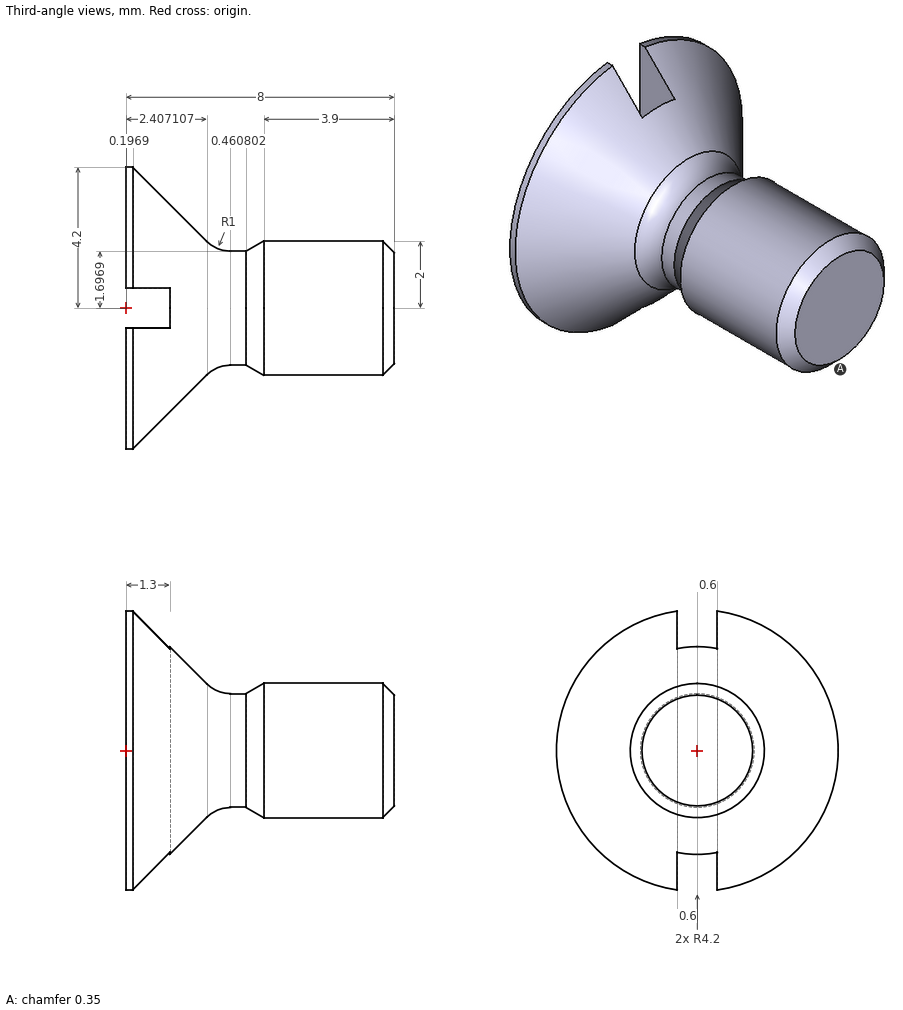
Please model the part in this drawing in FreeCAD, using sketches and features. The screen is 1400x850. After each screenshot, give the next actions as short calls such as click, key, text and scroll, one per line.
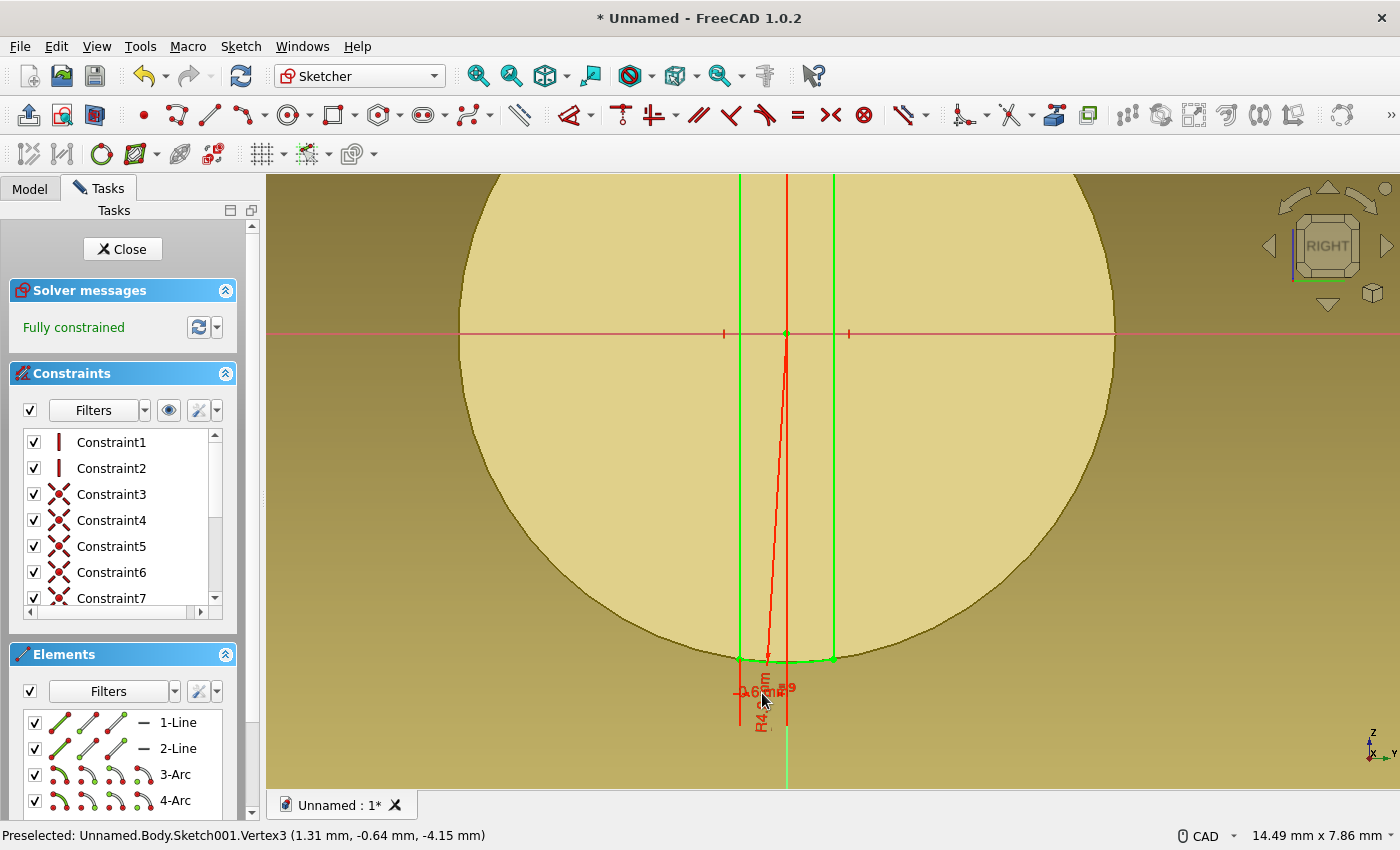
click(123, 249)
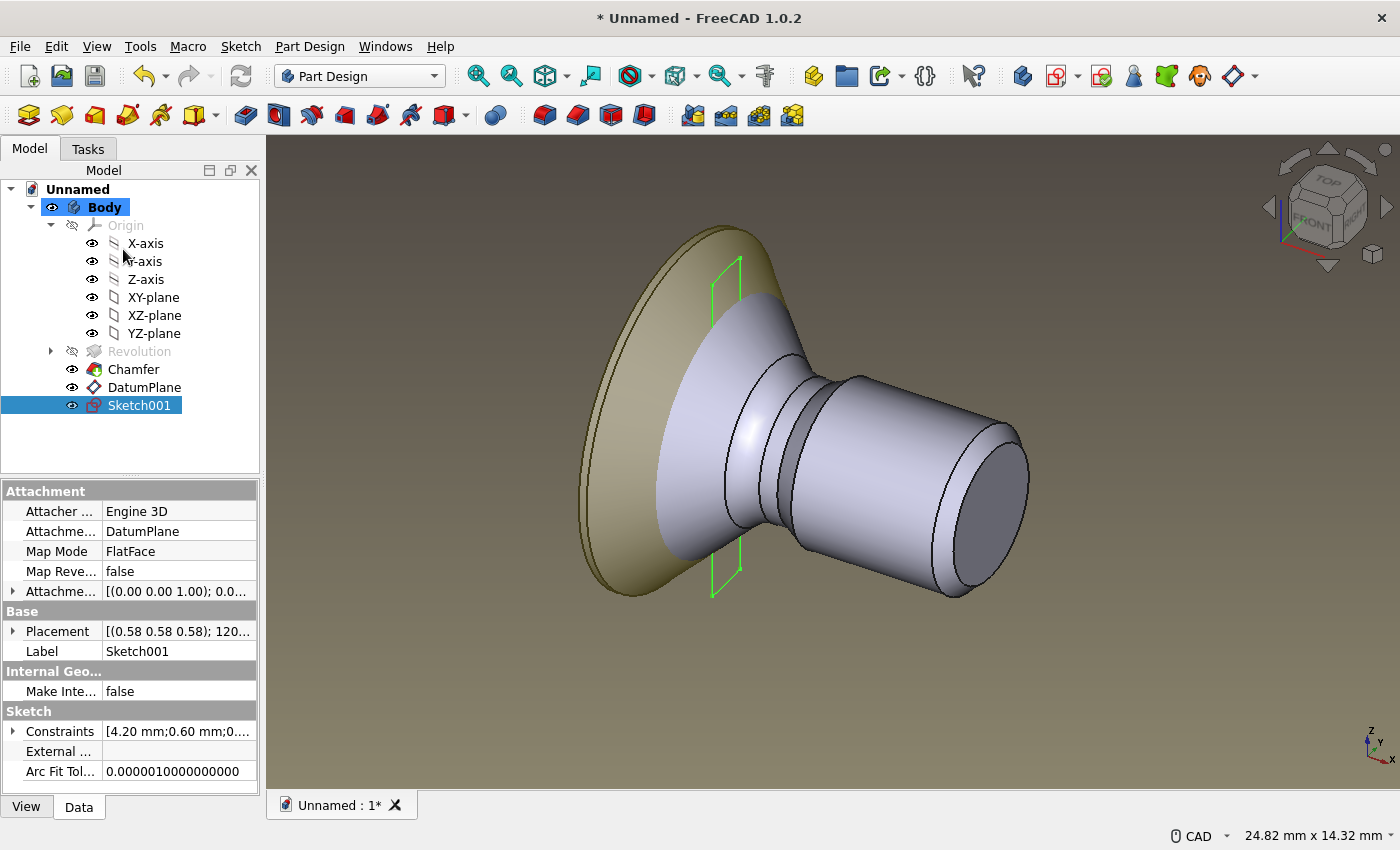
click(246, 116)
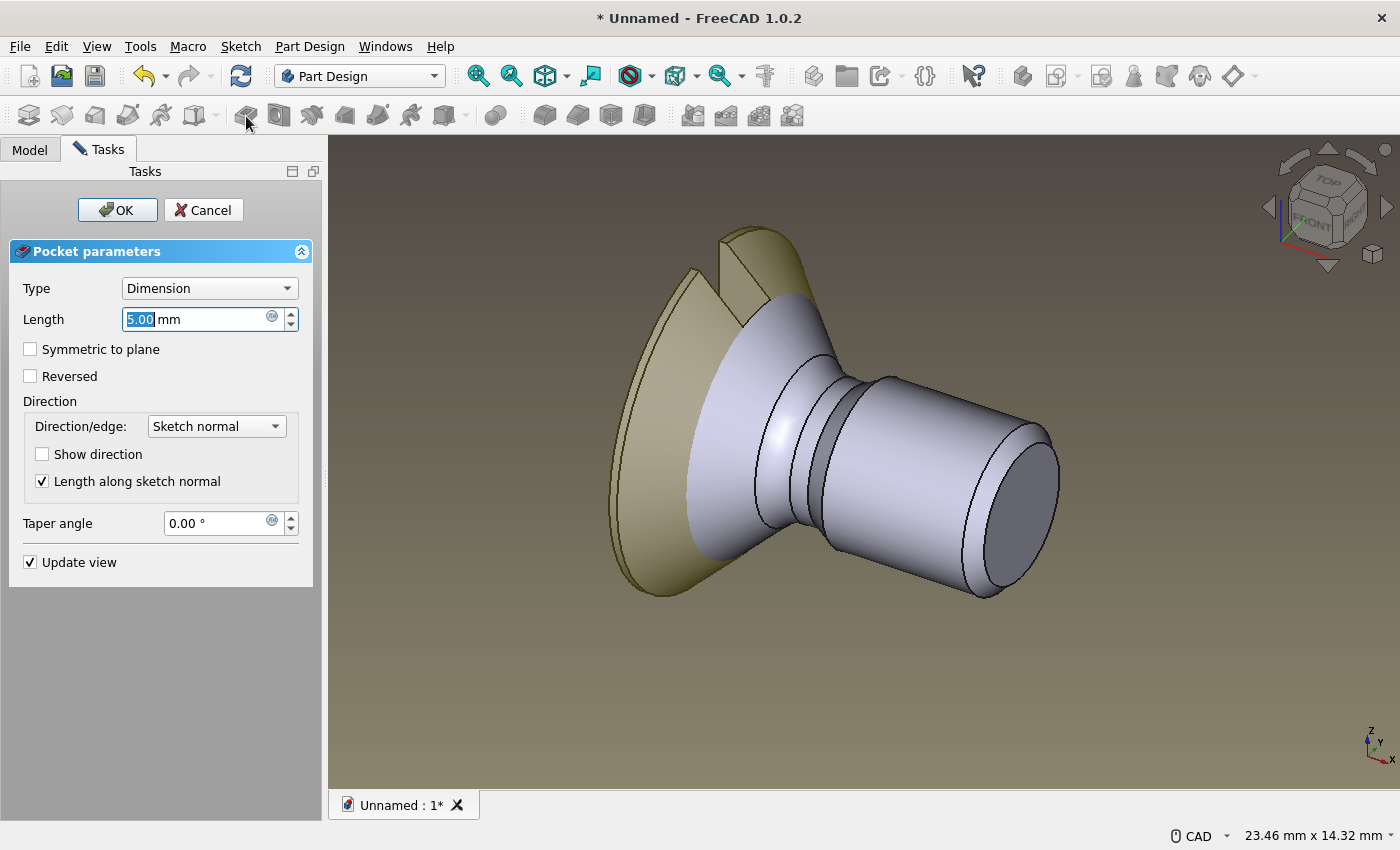
text(1.3)
key(Tab)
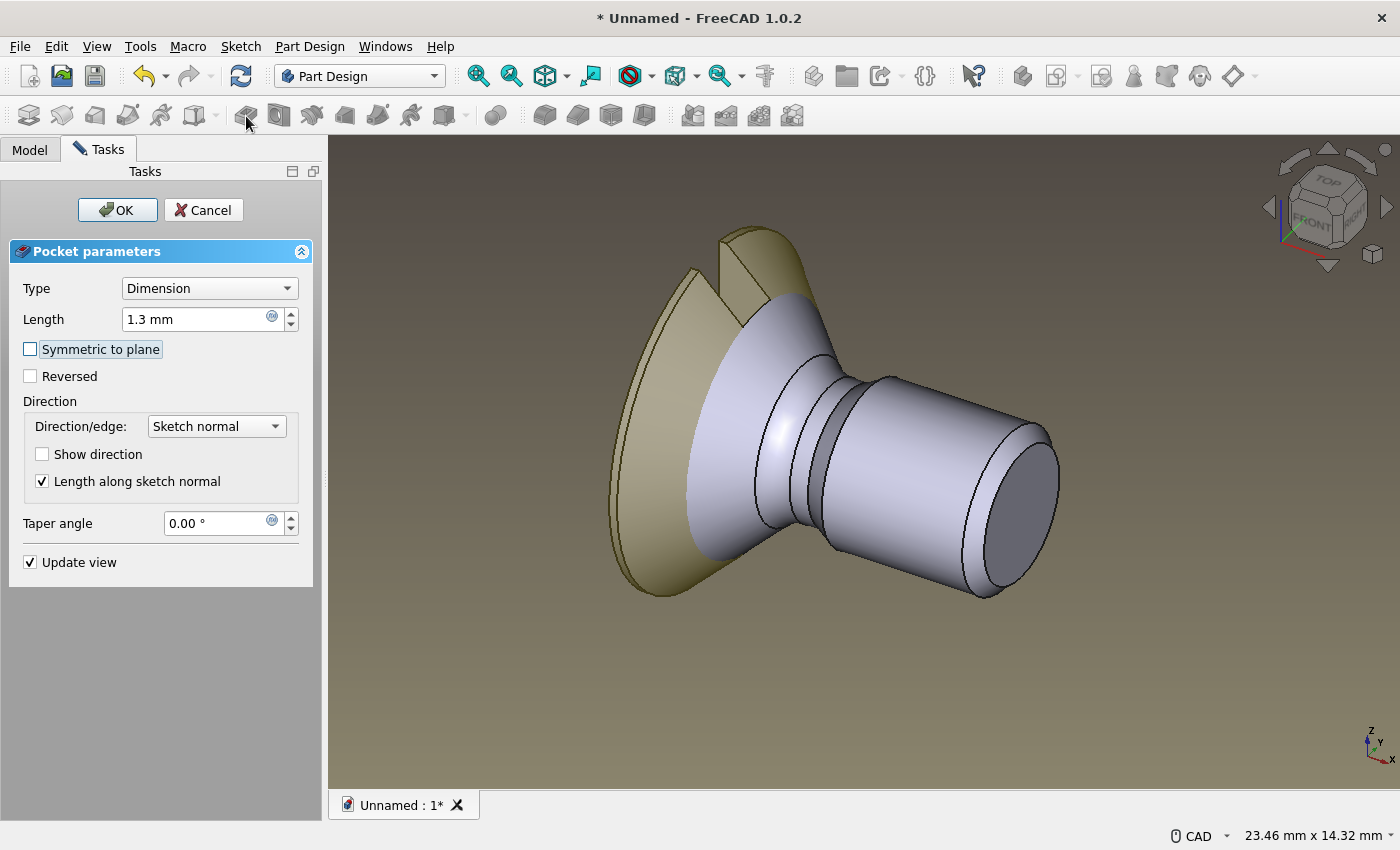
click(118, 210)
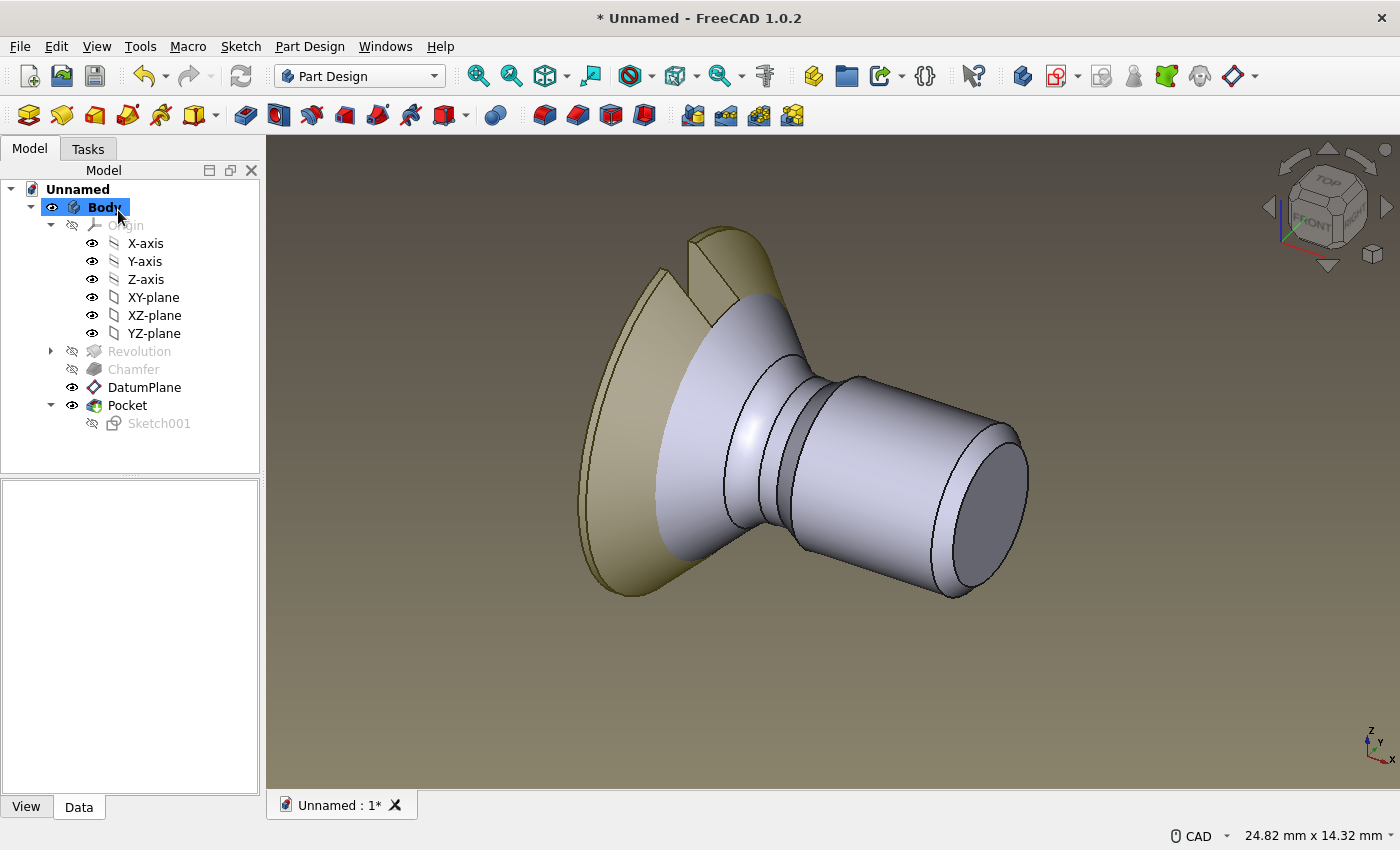
click(117, 387)
key(space)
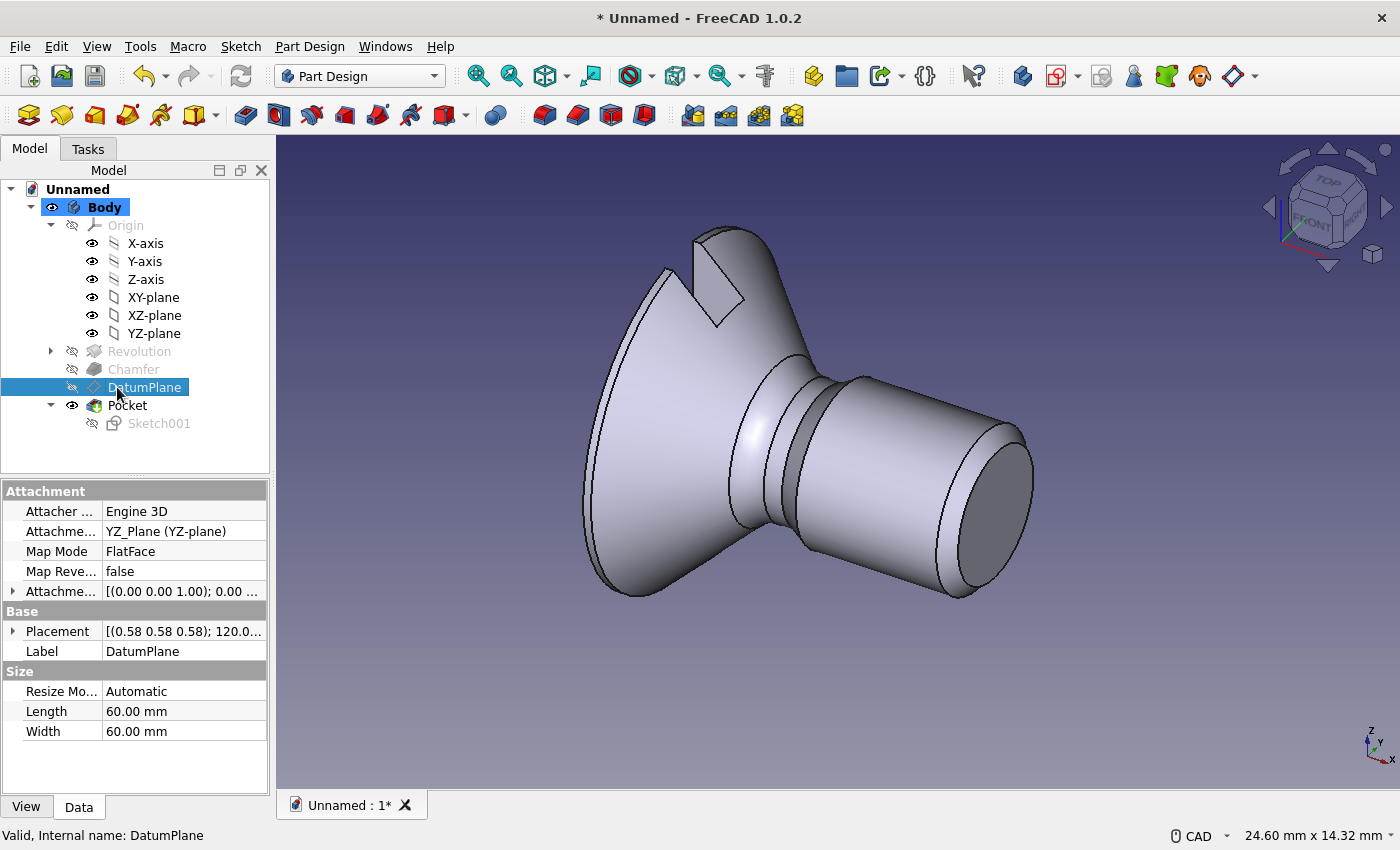
key(0)